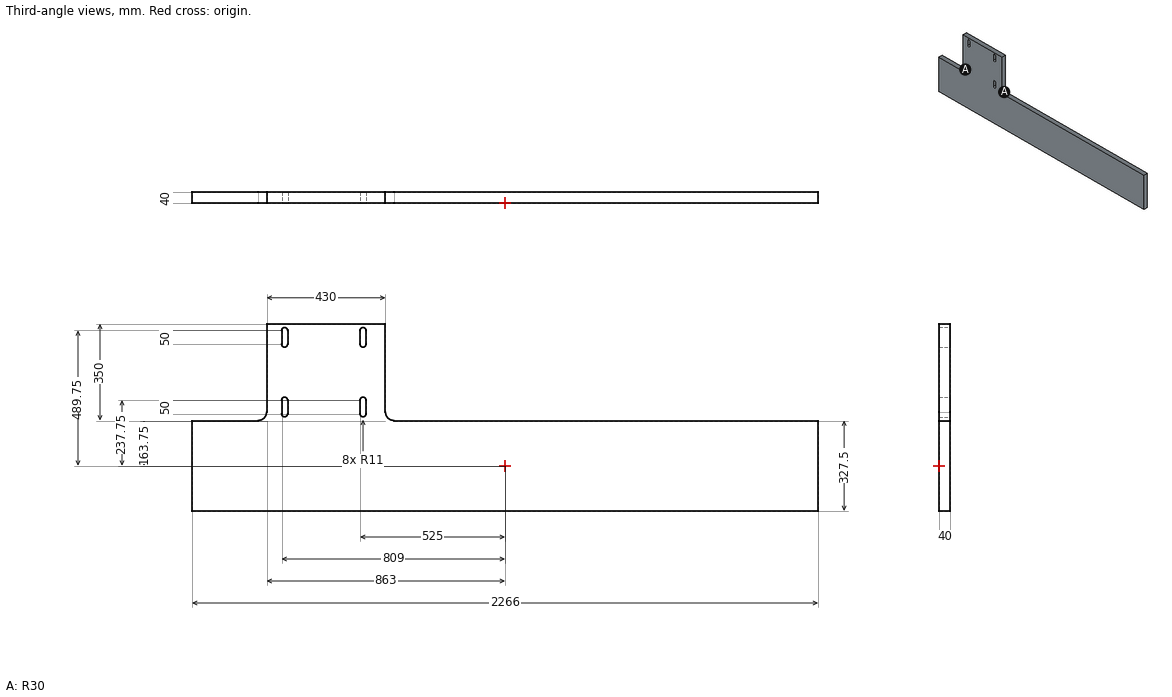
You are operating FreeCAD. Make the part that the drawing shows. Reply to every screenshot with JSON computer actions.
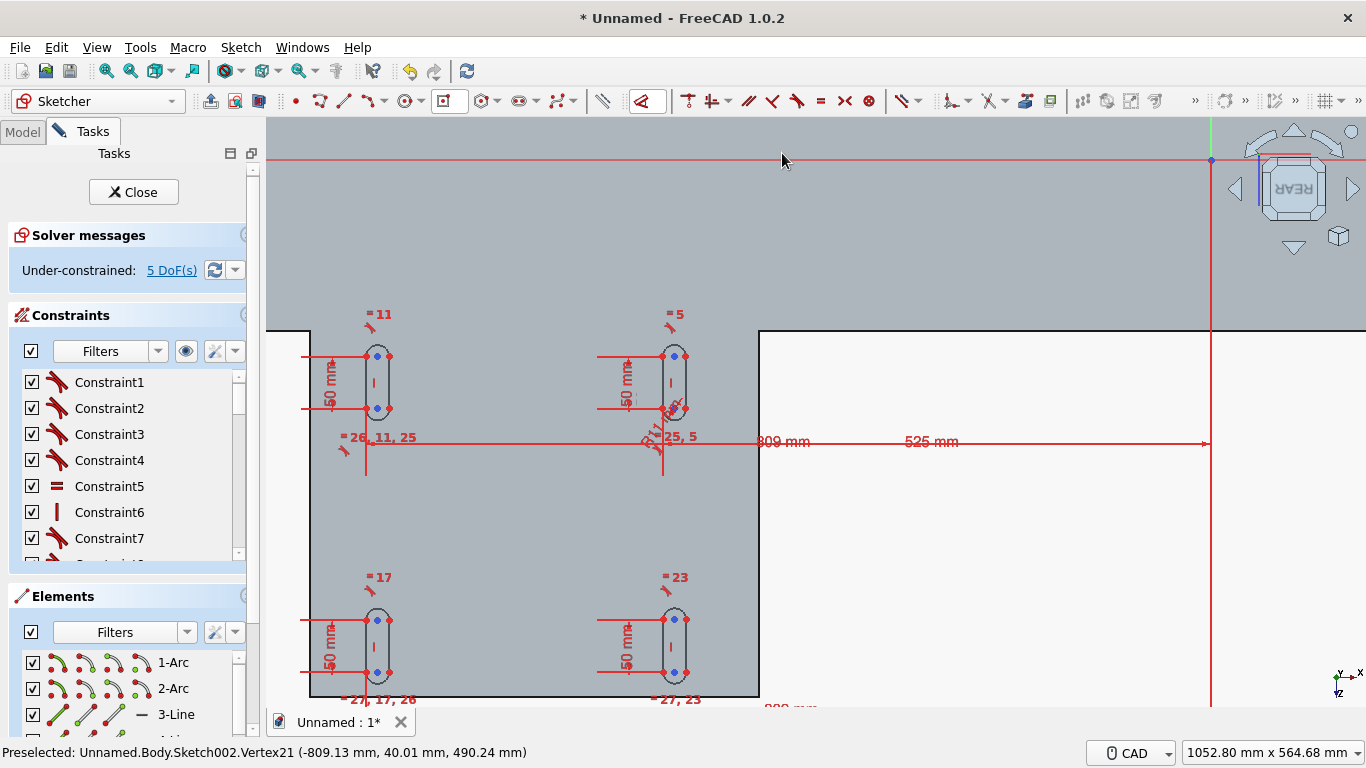
{"action": "left_click", "coordinate": [663, 672]}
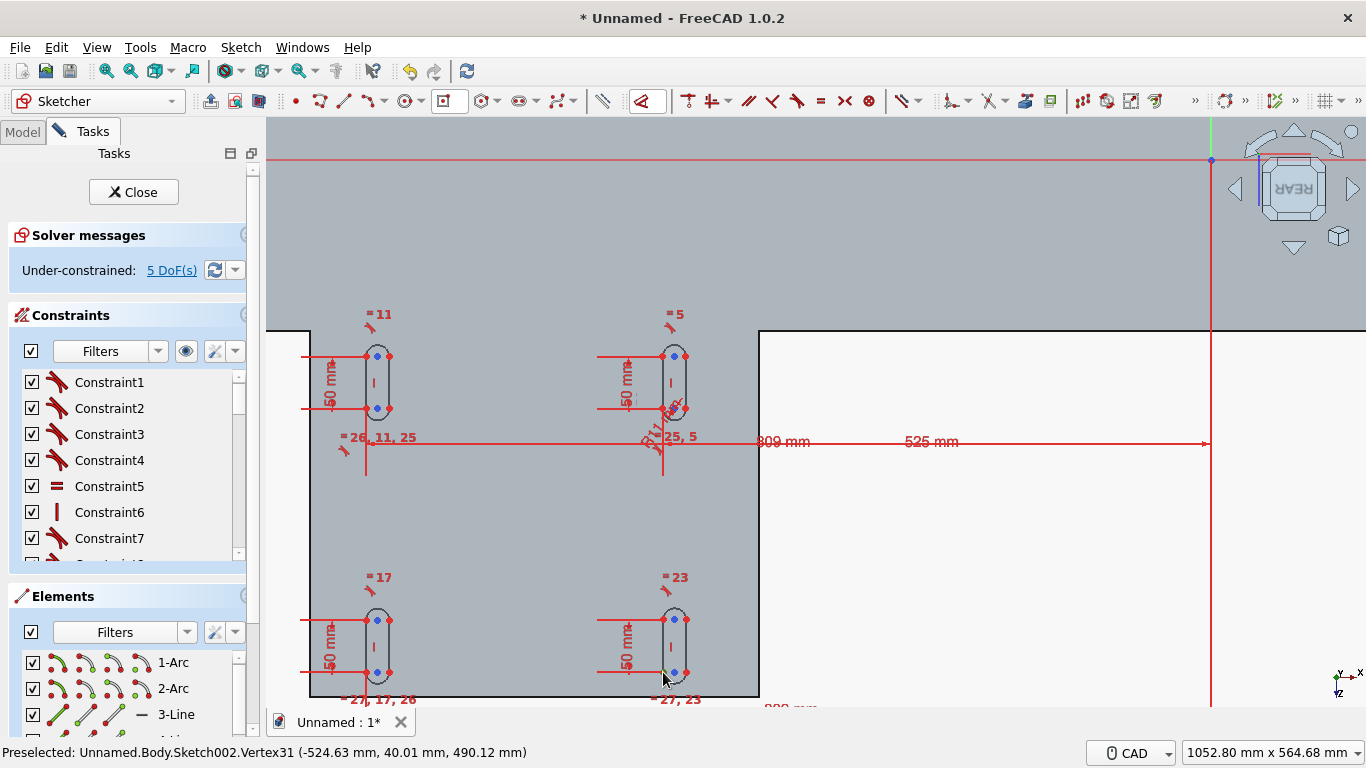
{"action": "key", "text": "l"}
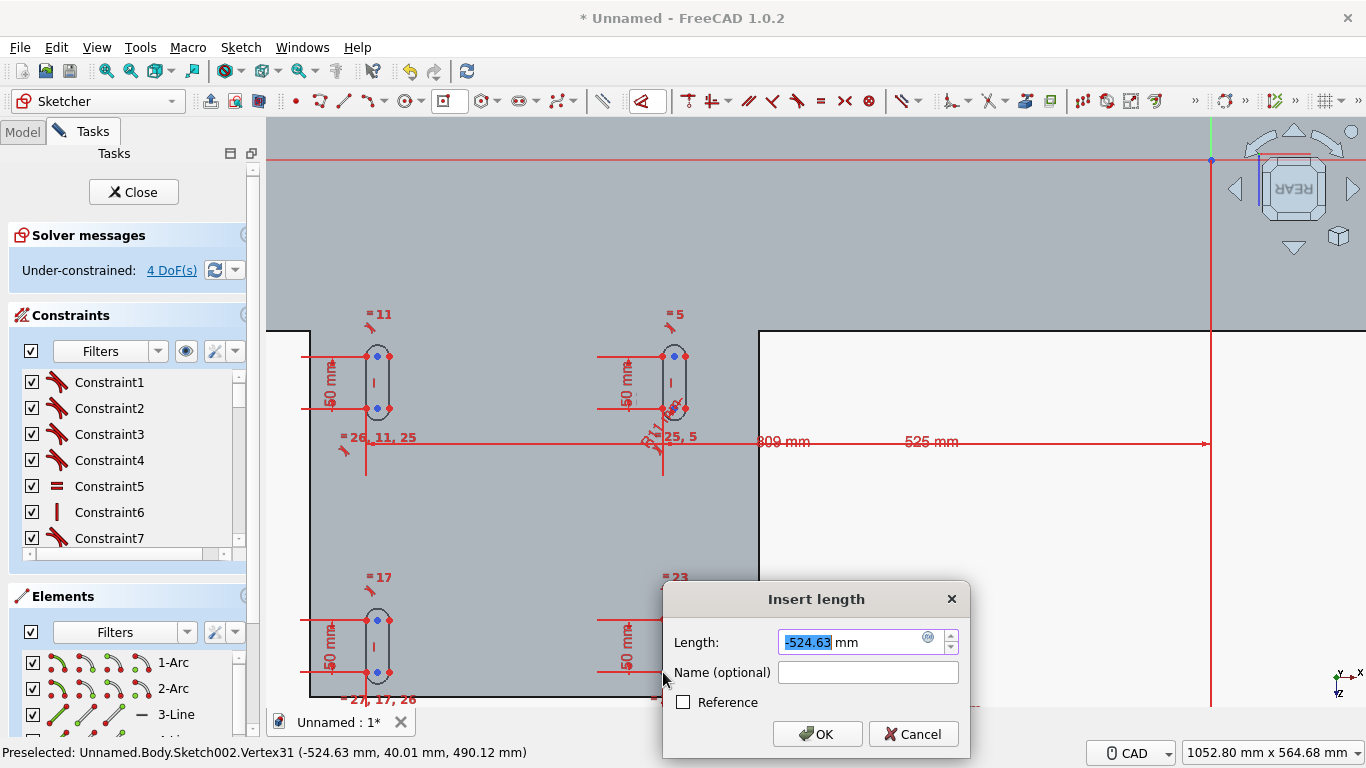
{"action": "type", "text": "-525"}
{"action": "key", "text": "Return"}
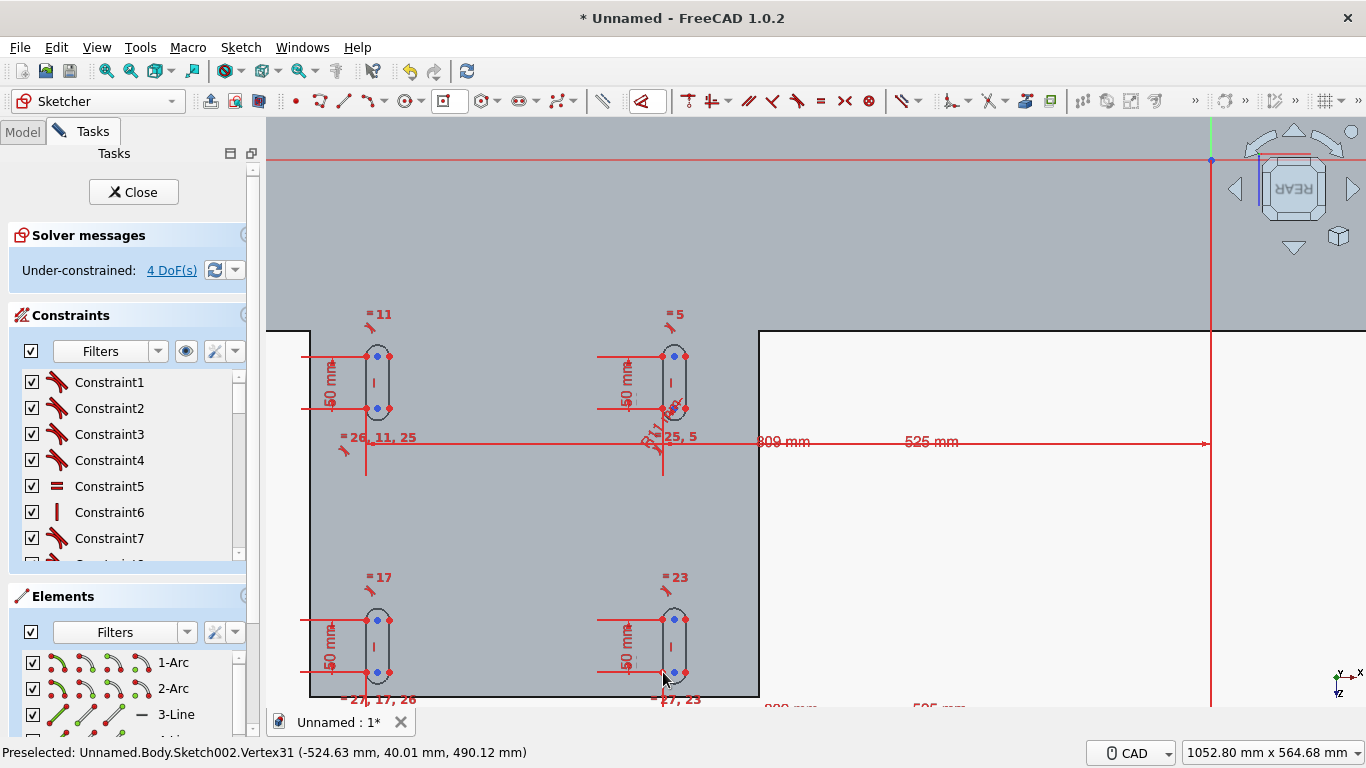
{"action": "left_click", "coordinate": [663, 409]}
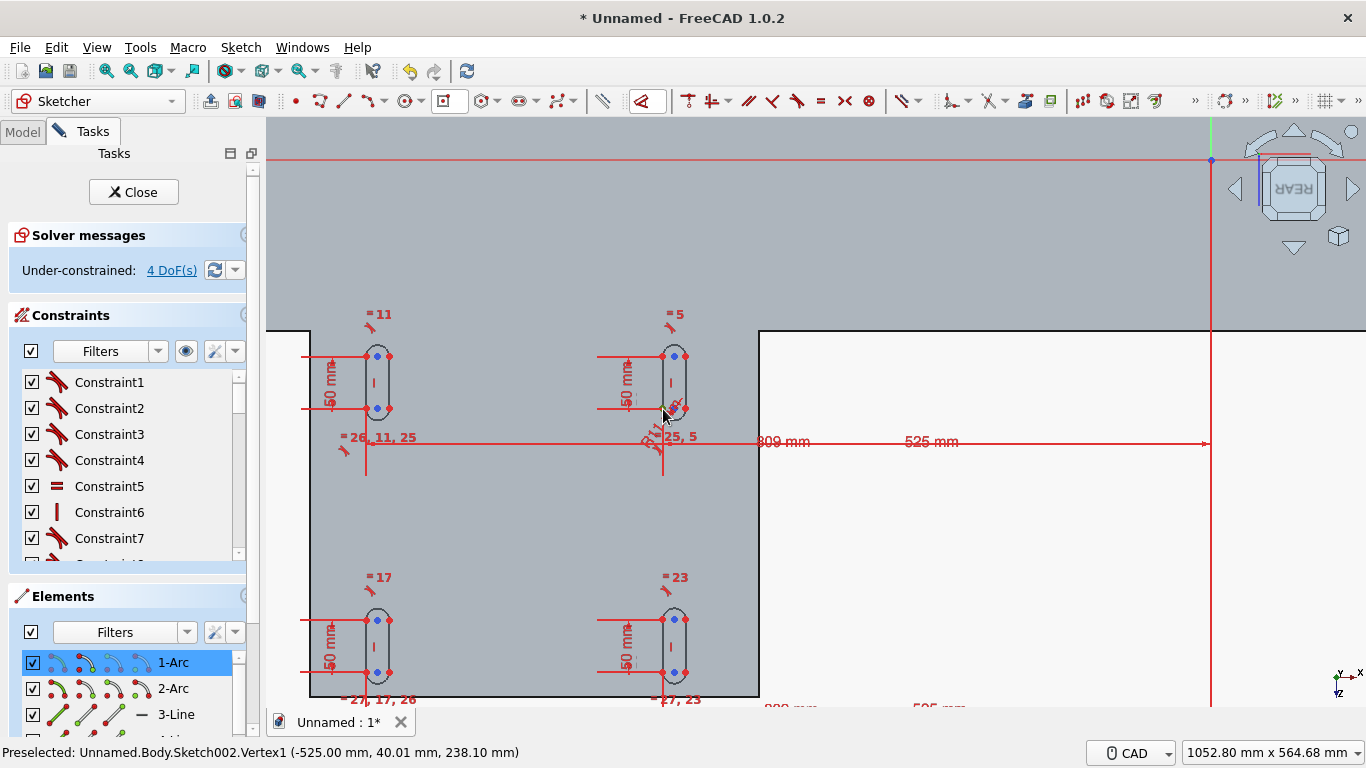
{"action": "key", "text": "i"}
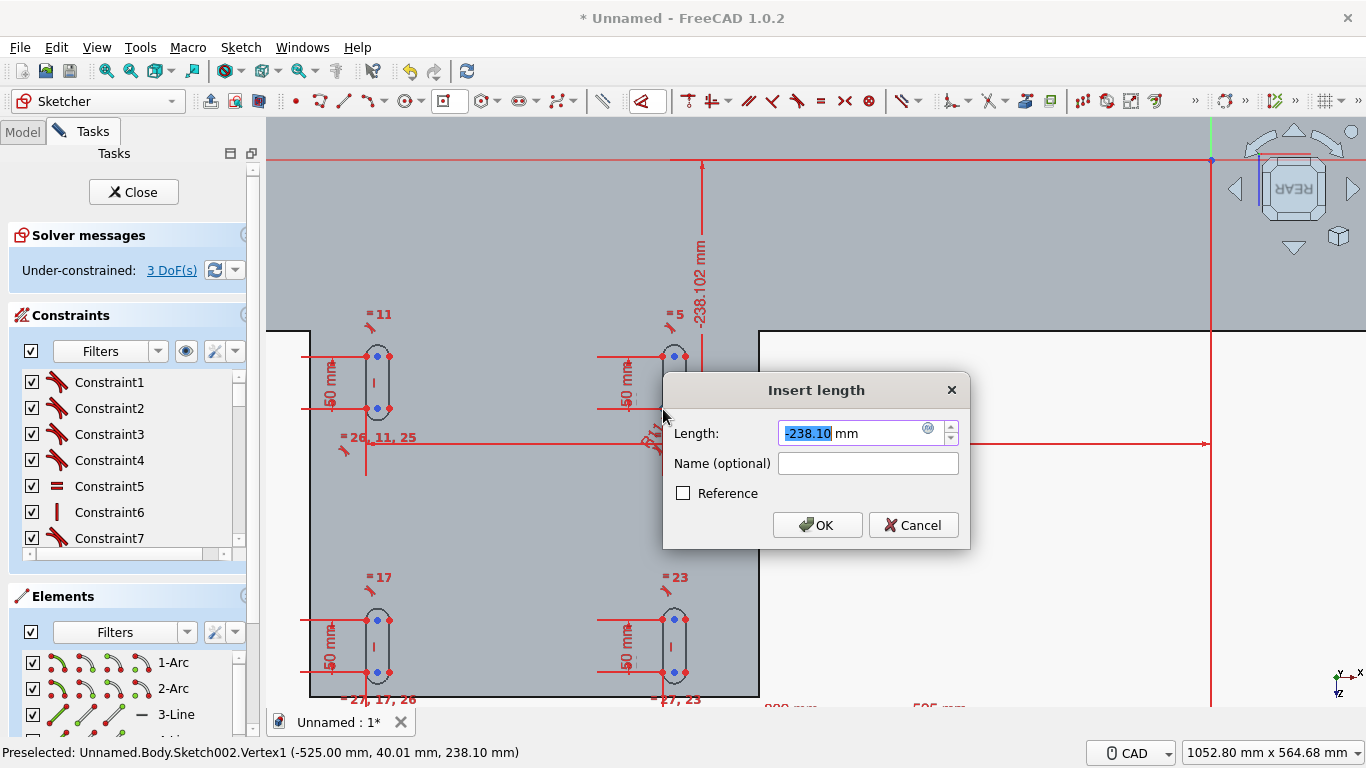
{"action": "type", "text": "-237.75"}
{"action": "key", "text": "Return"}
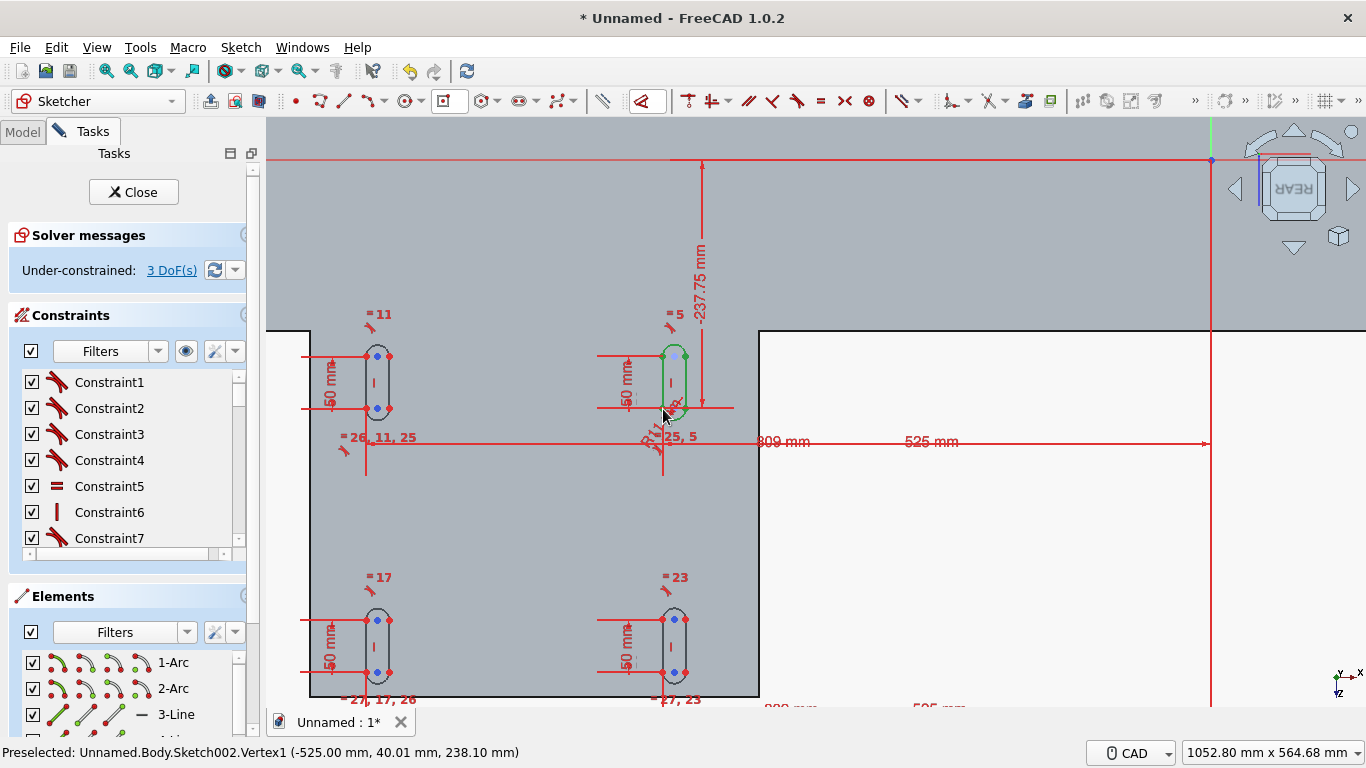
{"action": "left_click", "coordinate": [366, 409]}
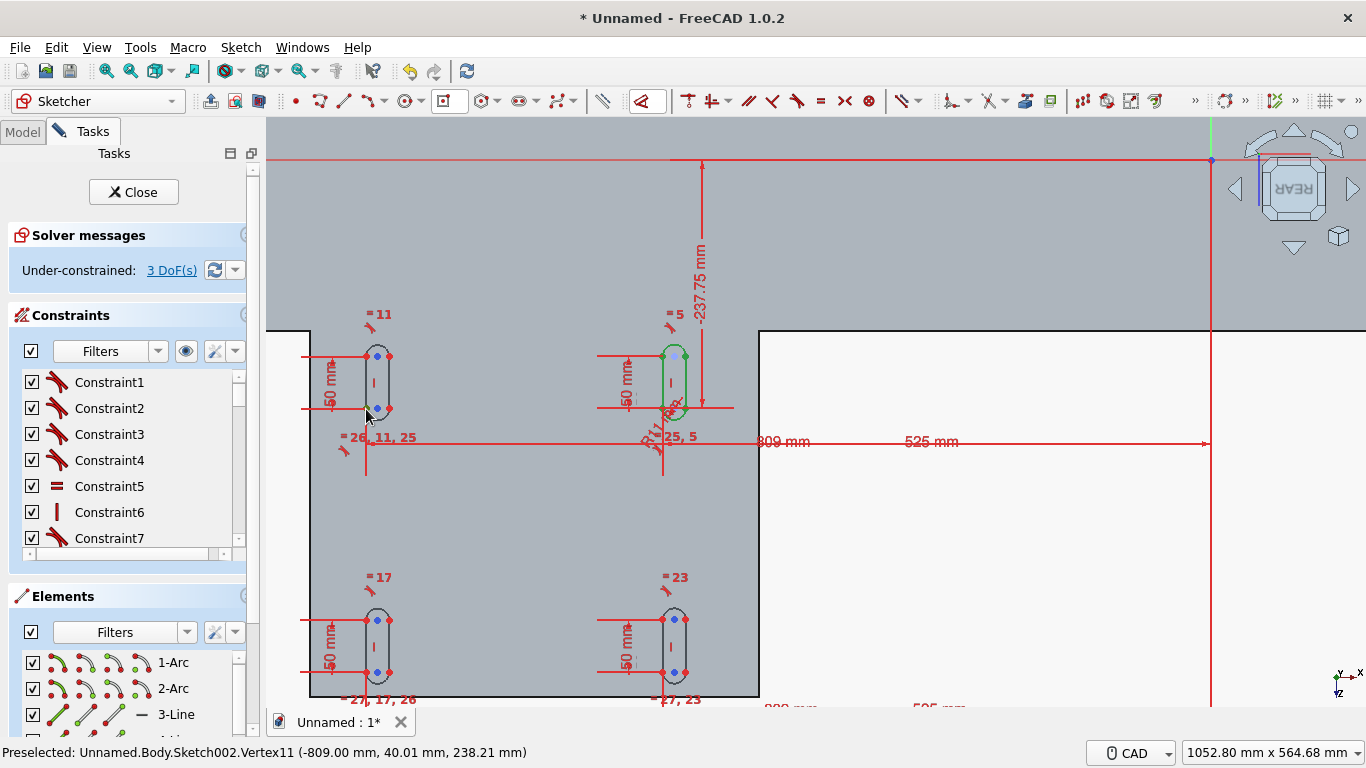
{"action": "left_click", "coordinate": [660, 102]}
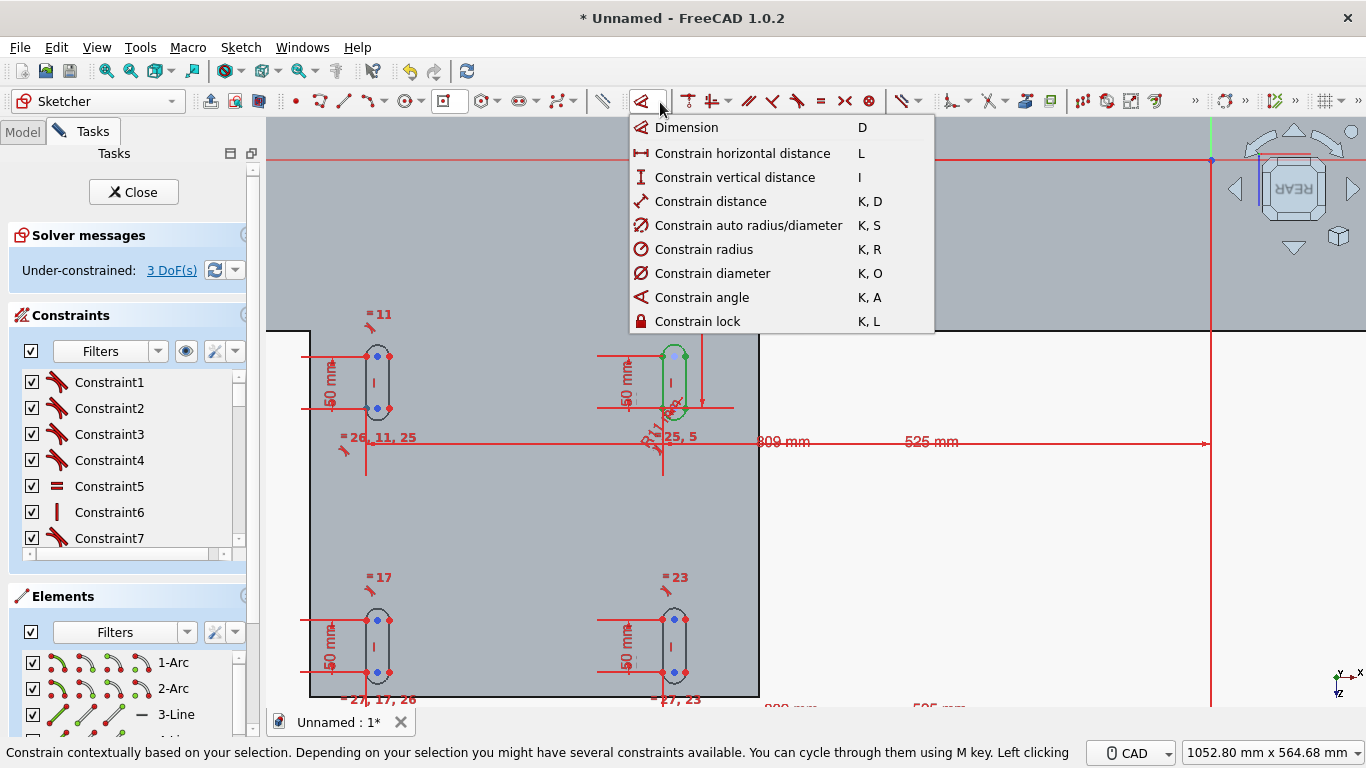
{"action": "left_click", "coordinate": [782, 177]}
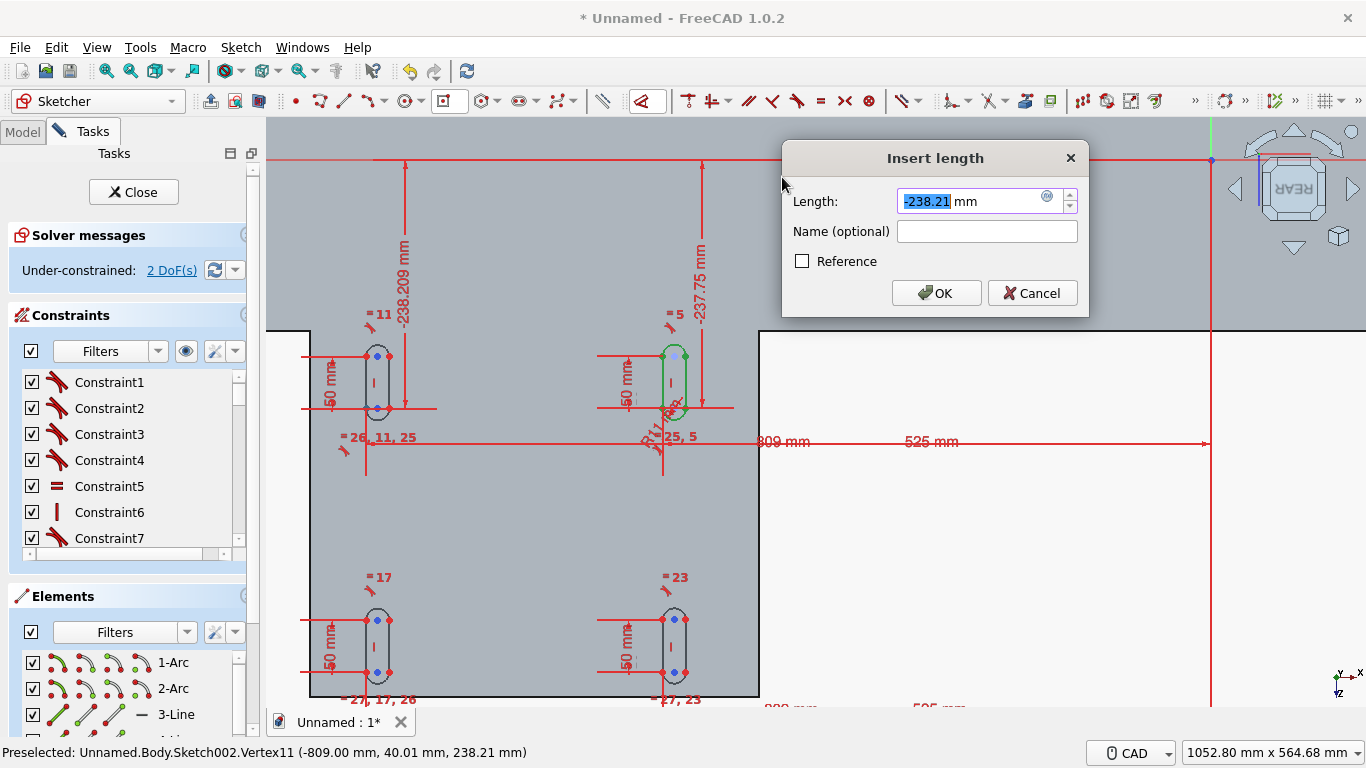
{"action": "type", "text": "-237.75"}
{"action": "key", "text": "Return"}